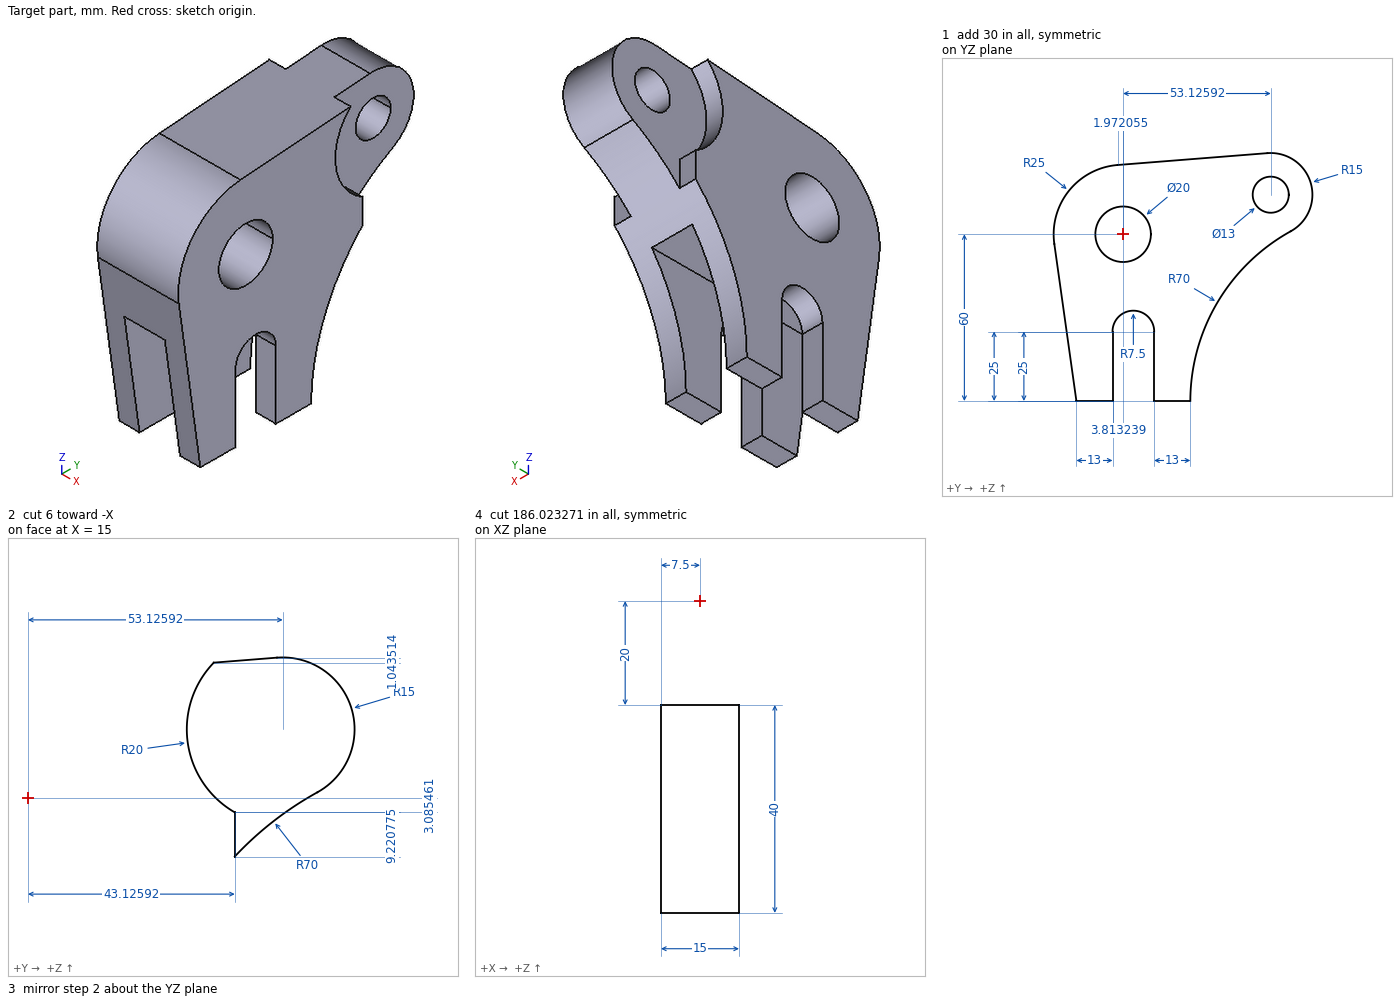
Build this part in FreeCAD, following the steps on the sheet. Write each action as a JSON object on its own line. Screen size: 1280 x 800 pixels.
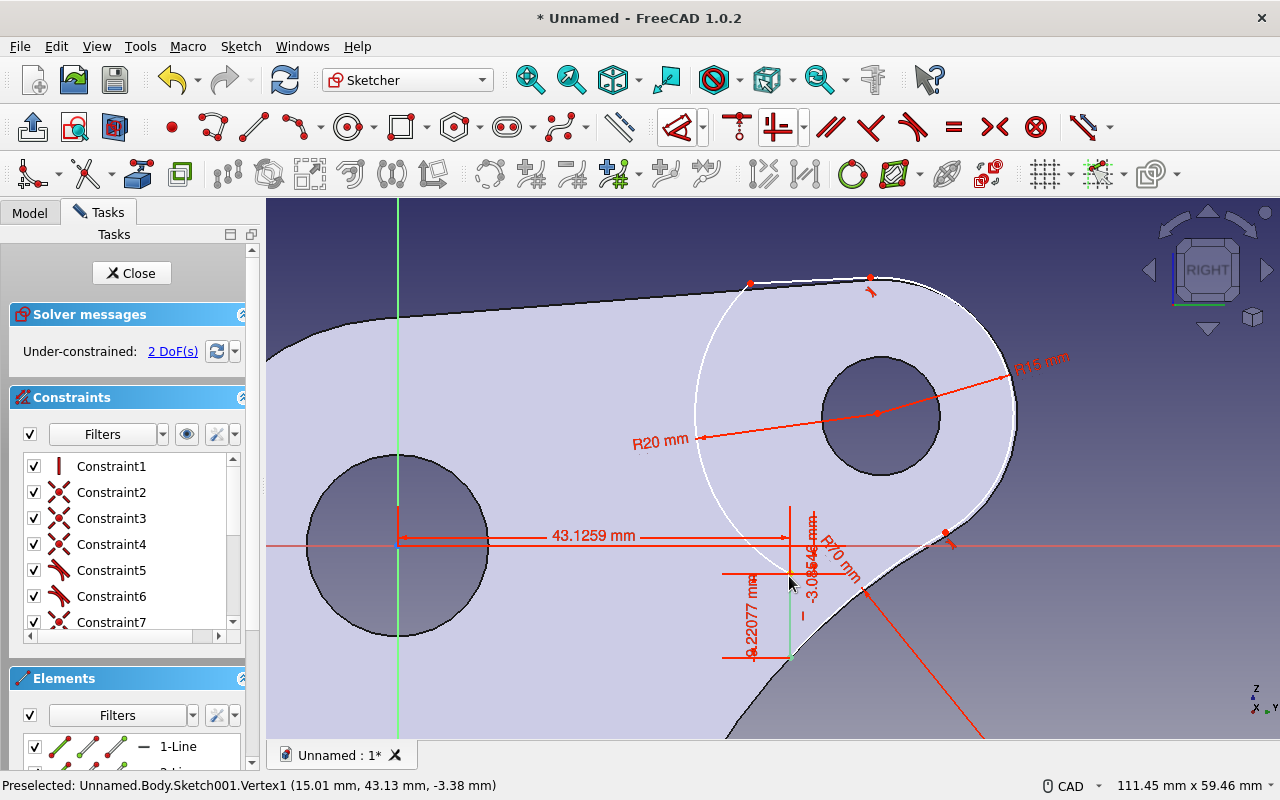
{"action": "scroll", "coordinate": [834, 279], "scroll_direction": "up", "scroll_amount": 8}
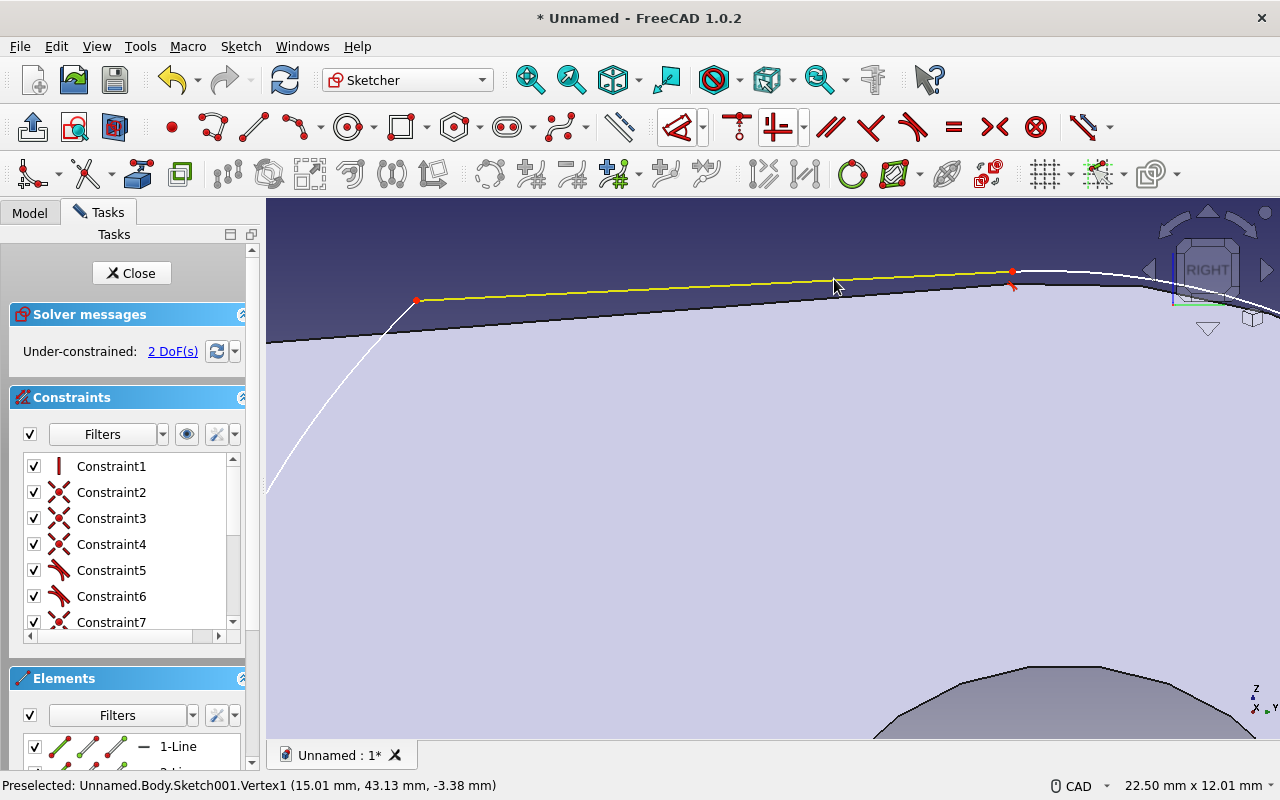
{"action": "left_click", "coordinate": [834, 280]}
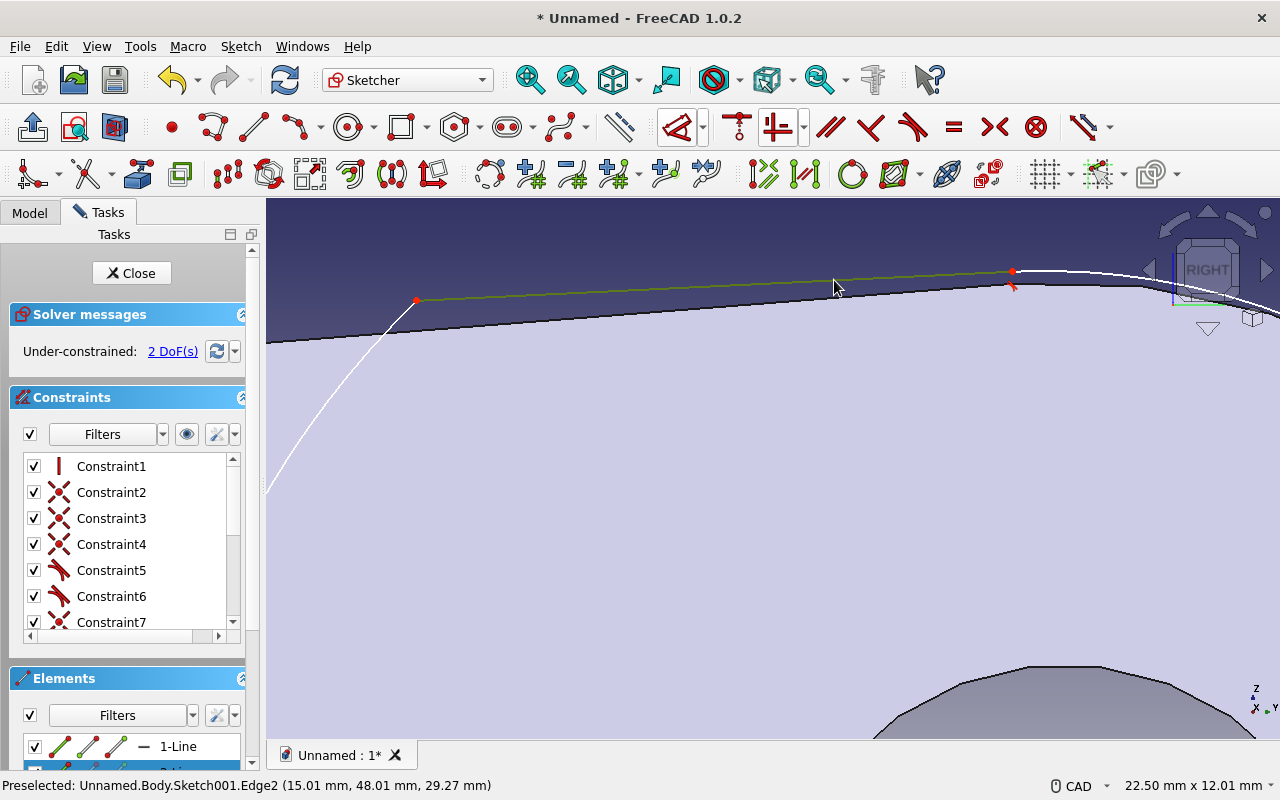
{"action": "left_click", "coordinate": [702, 128]}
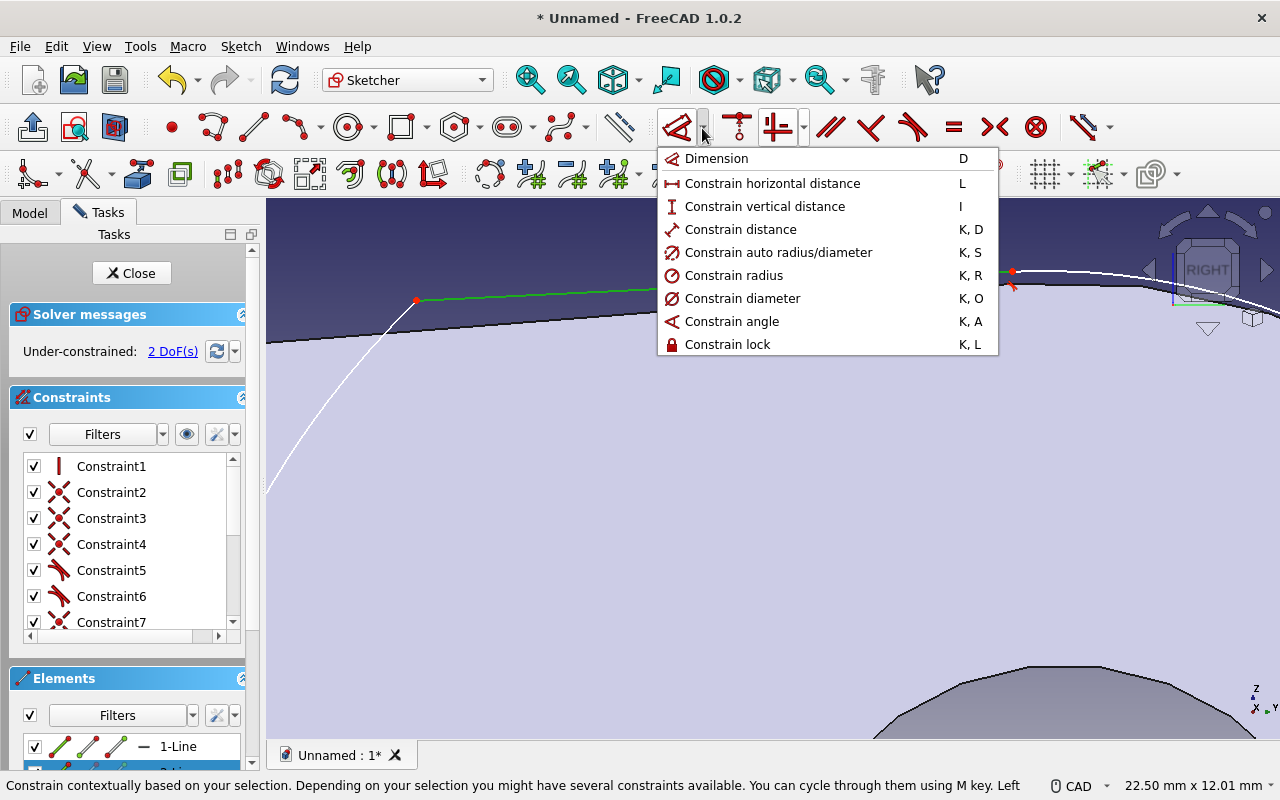
{"action": "left_click", "coordinate": [828, 206]}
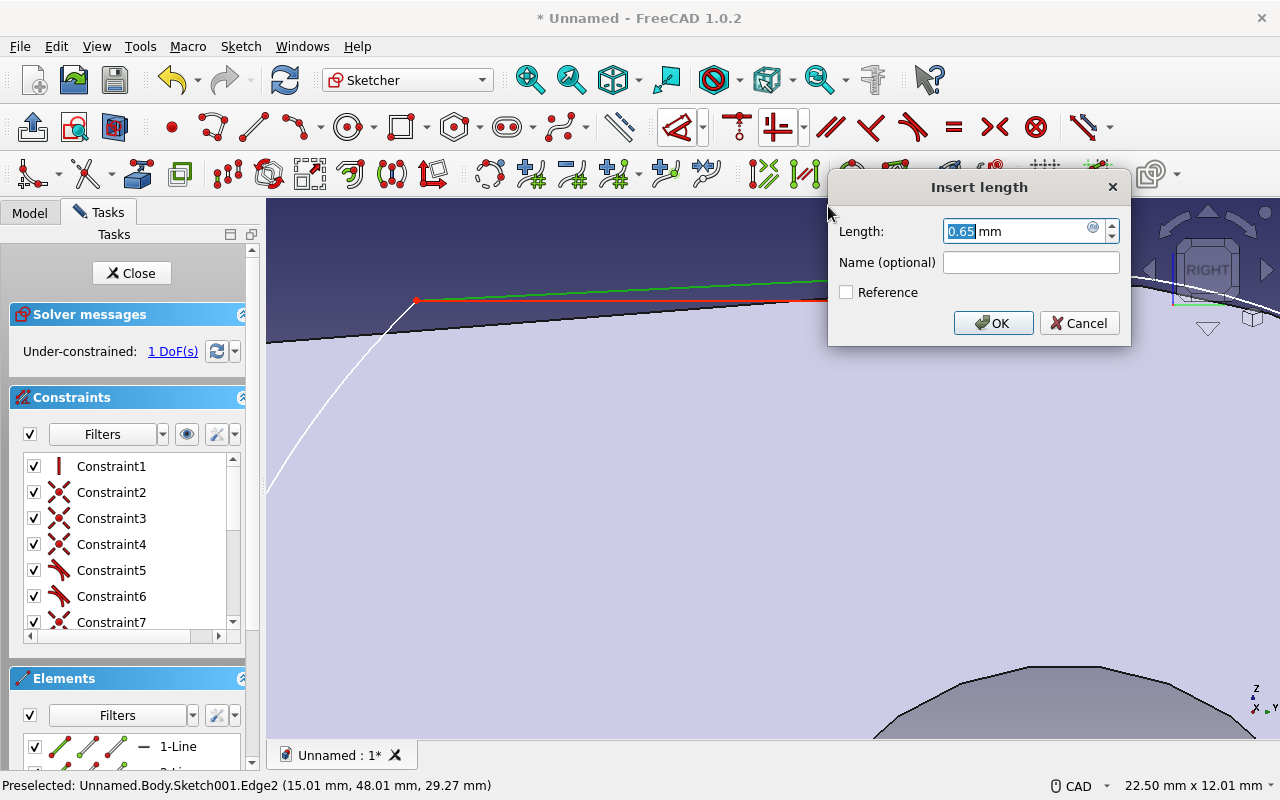
{"action": "type", "text": "1.043514"}
{"action": "key", "text": "Return"}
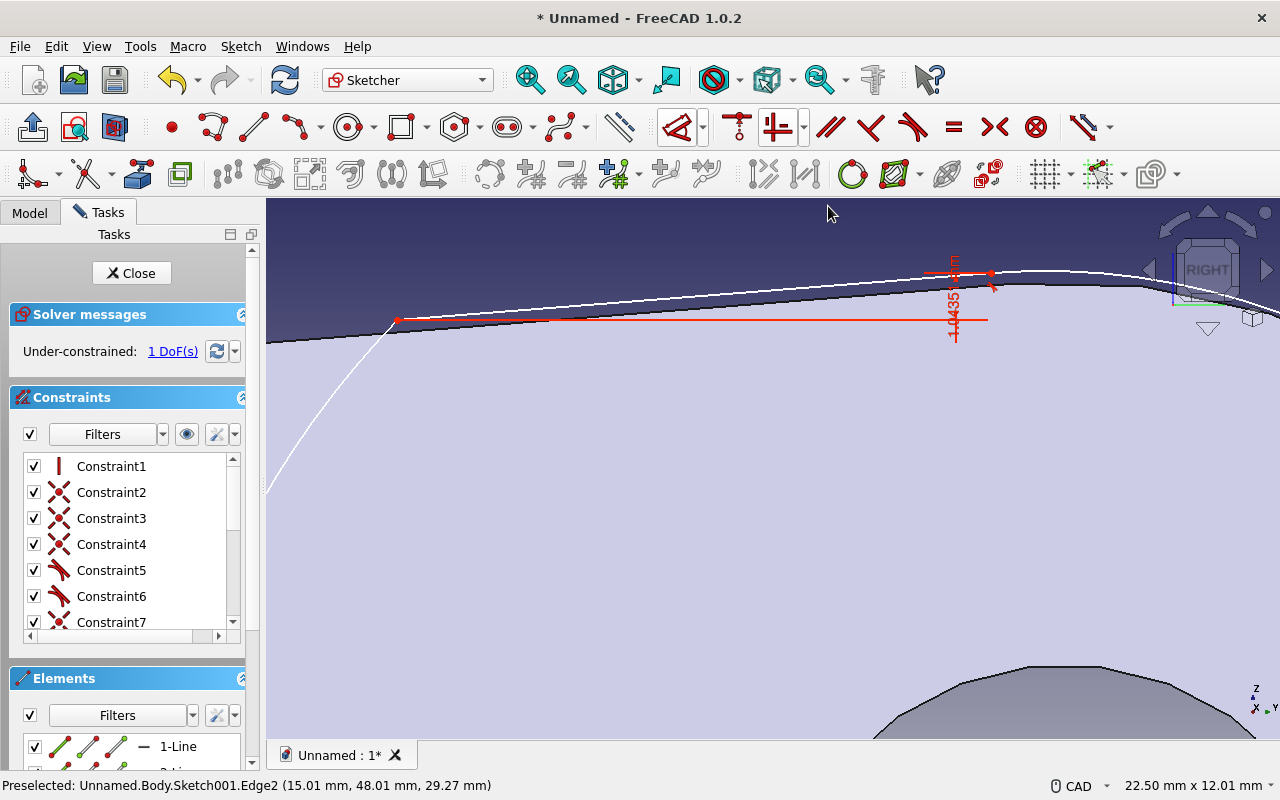
{"action": "scroll", "coordinate": [834, 279], "scroll_direction": "down", "scroll_amount": 8}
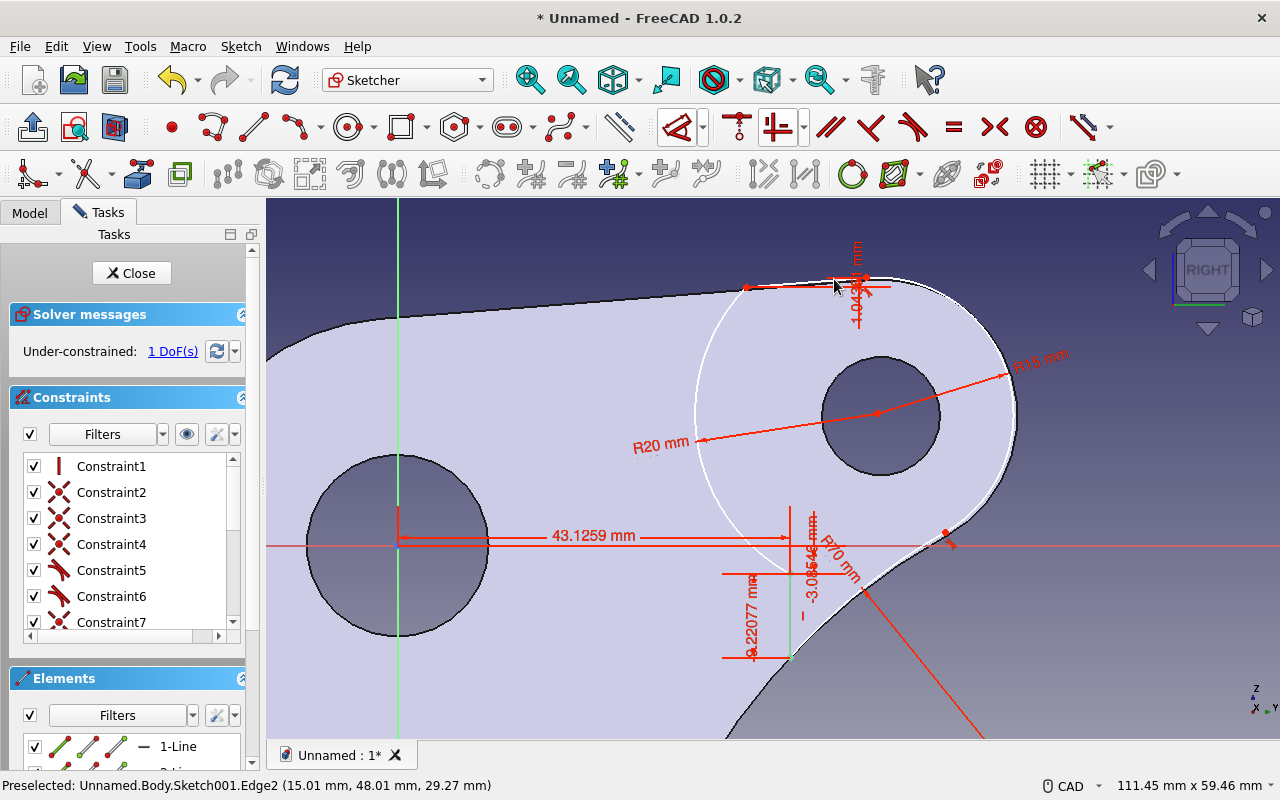
{"action": "left_click", "coordinate": [877, 414]}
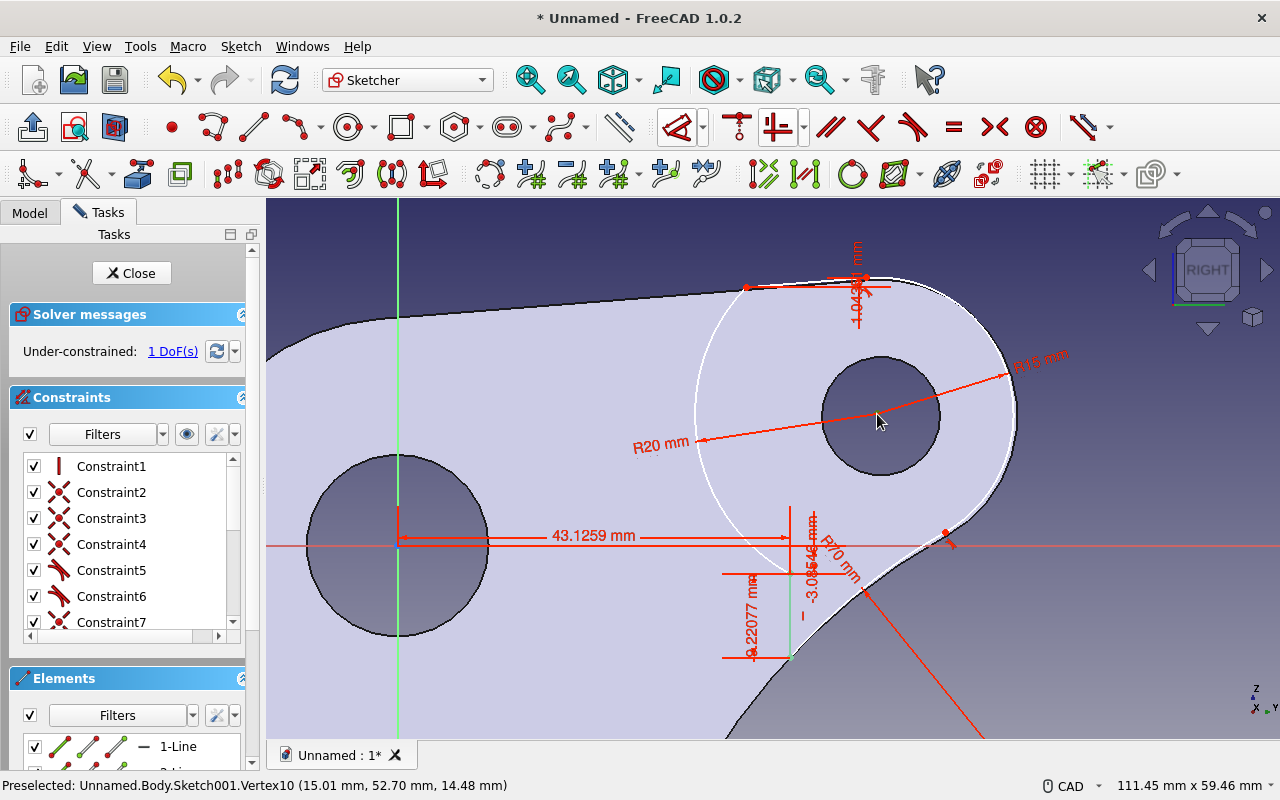
{"action": "key", "text": "l"}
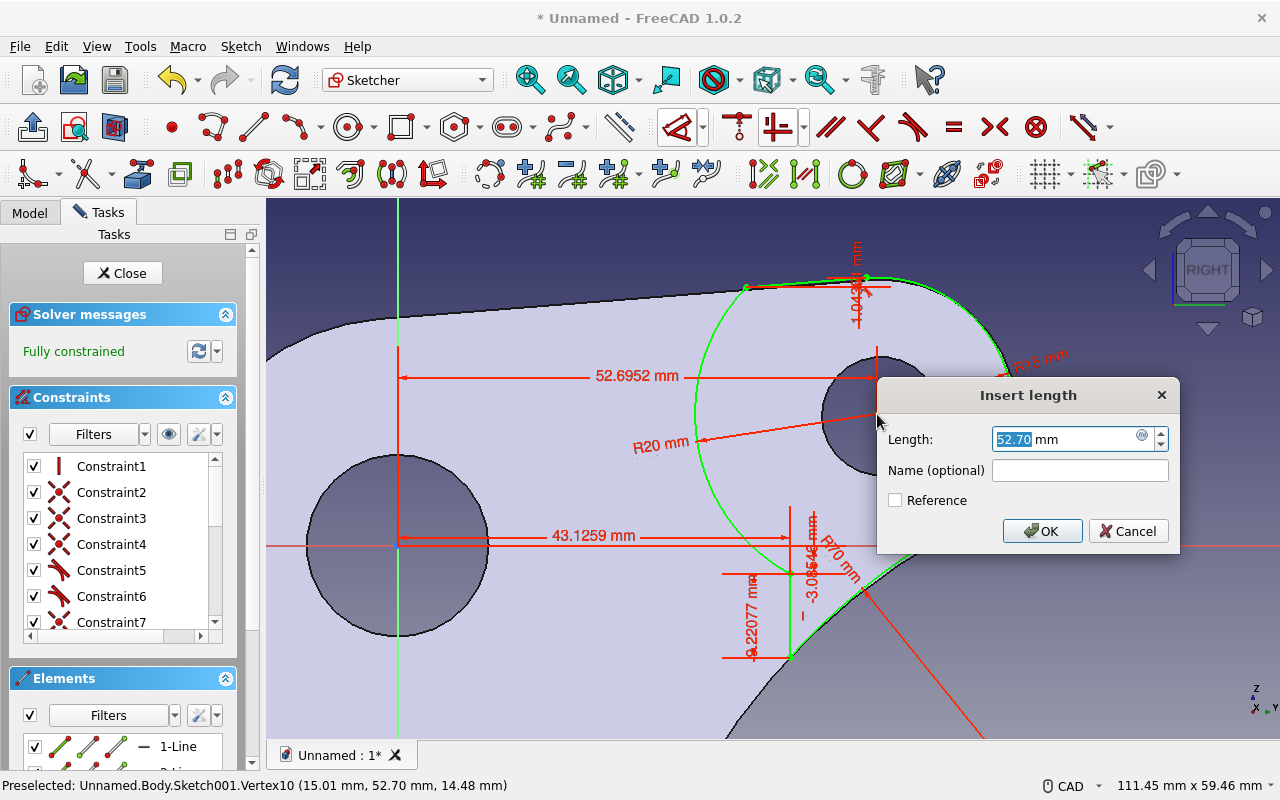
{"action": "type", "text": "53.12592"}
{"action": "key", "text": "Return"}